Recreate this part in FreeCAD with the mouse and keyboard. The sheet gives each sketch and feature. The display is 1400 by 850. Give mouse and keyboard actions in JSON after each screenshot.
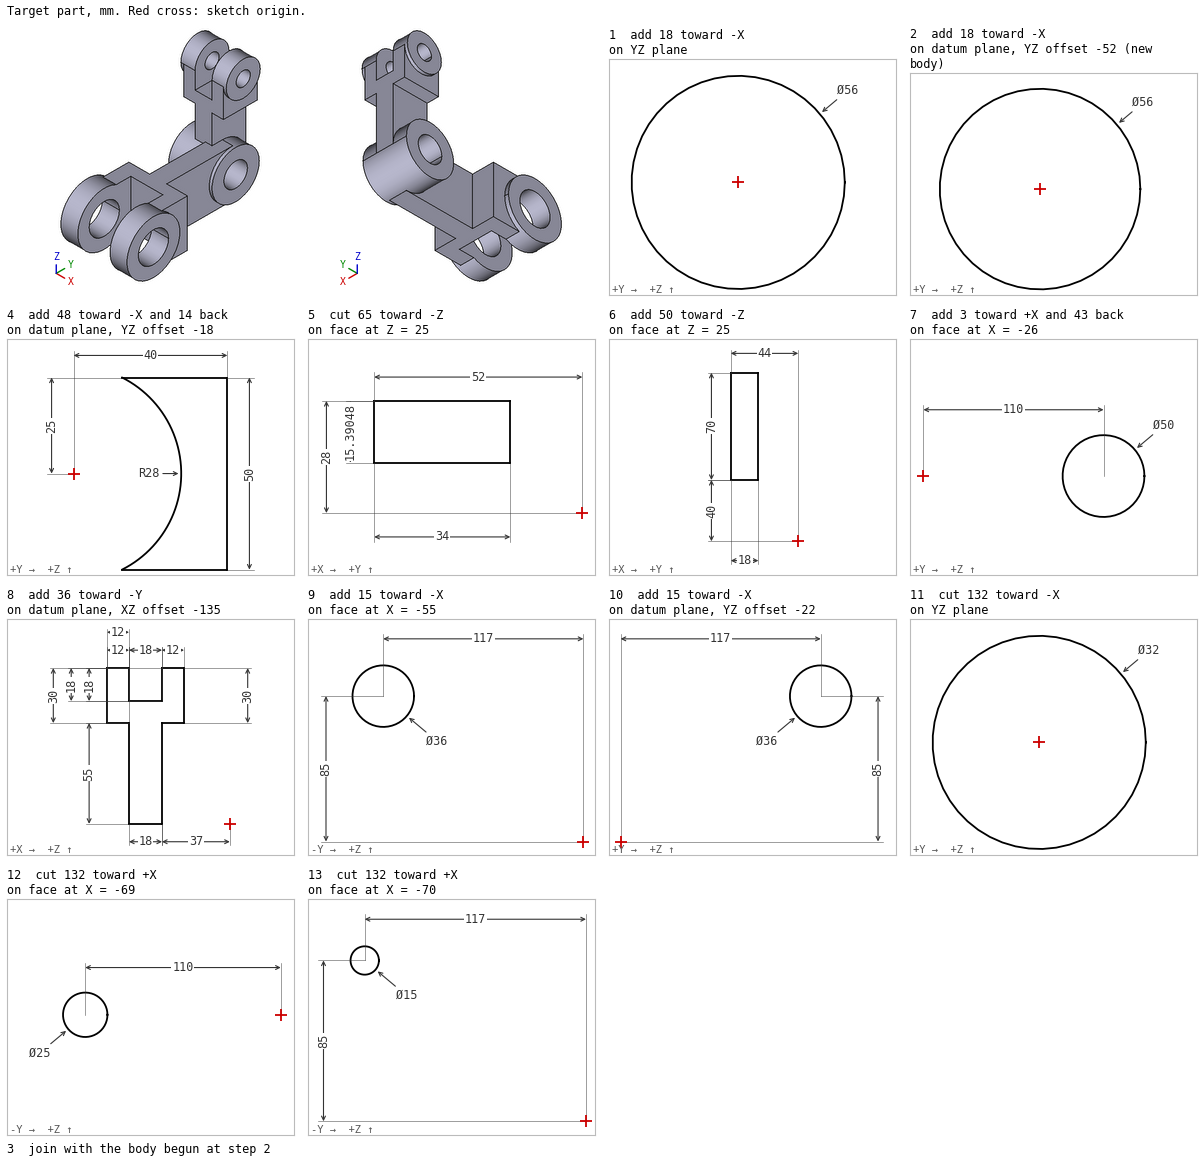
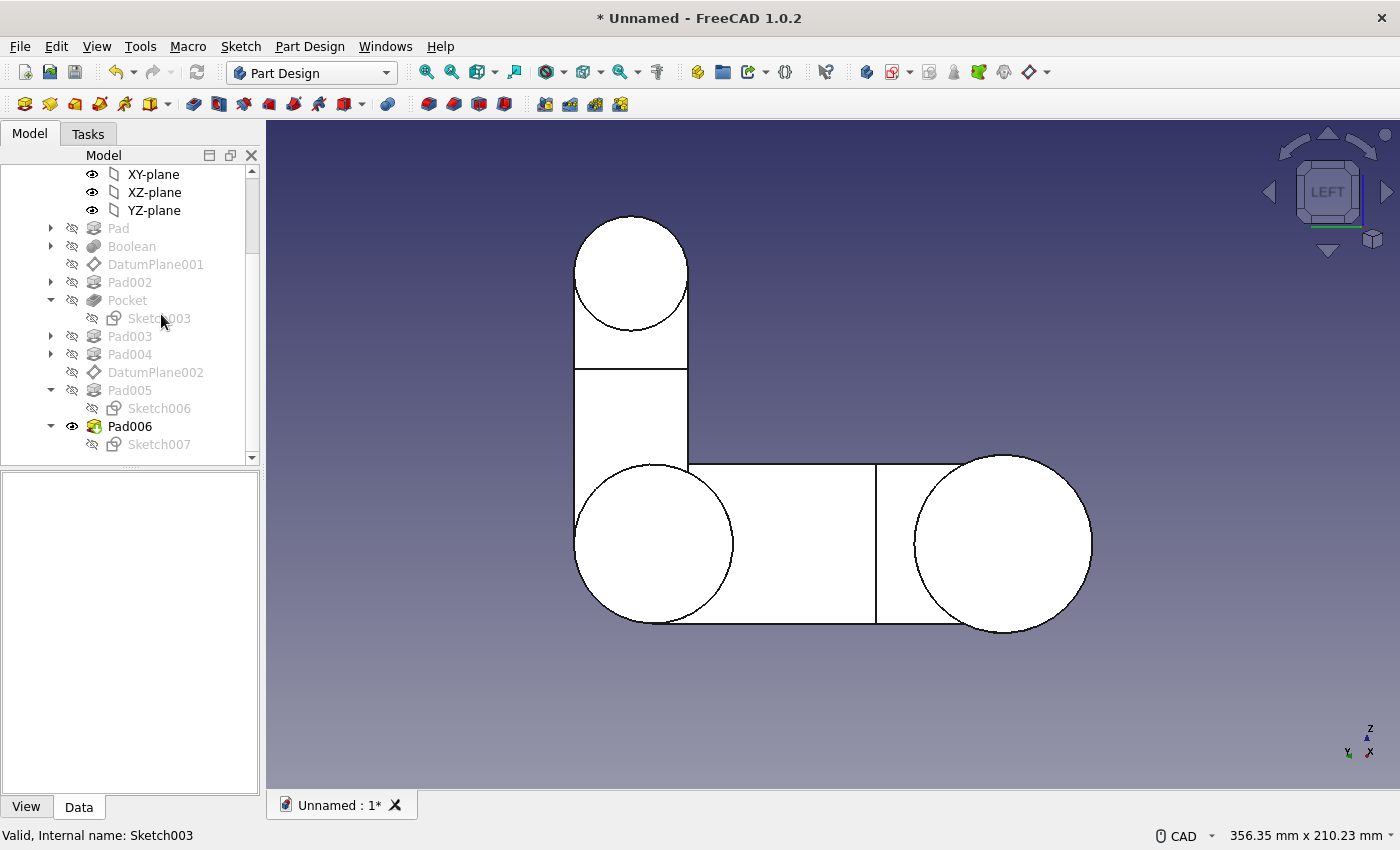
{"action": "scroll", "coordinate": [161, 314], "scroll_direction": "up", "scroll_amount": 15}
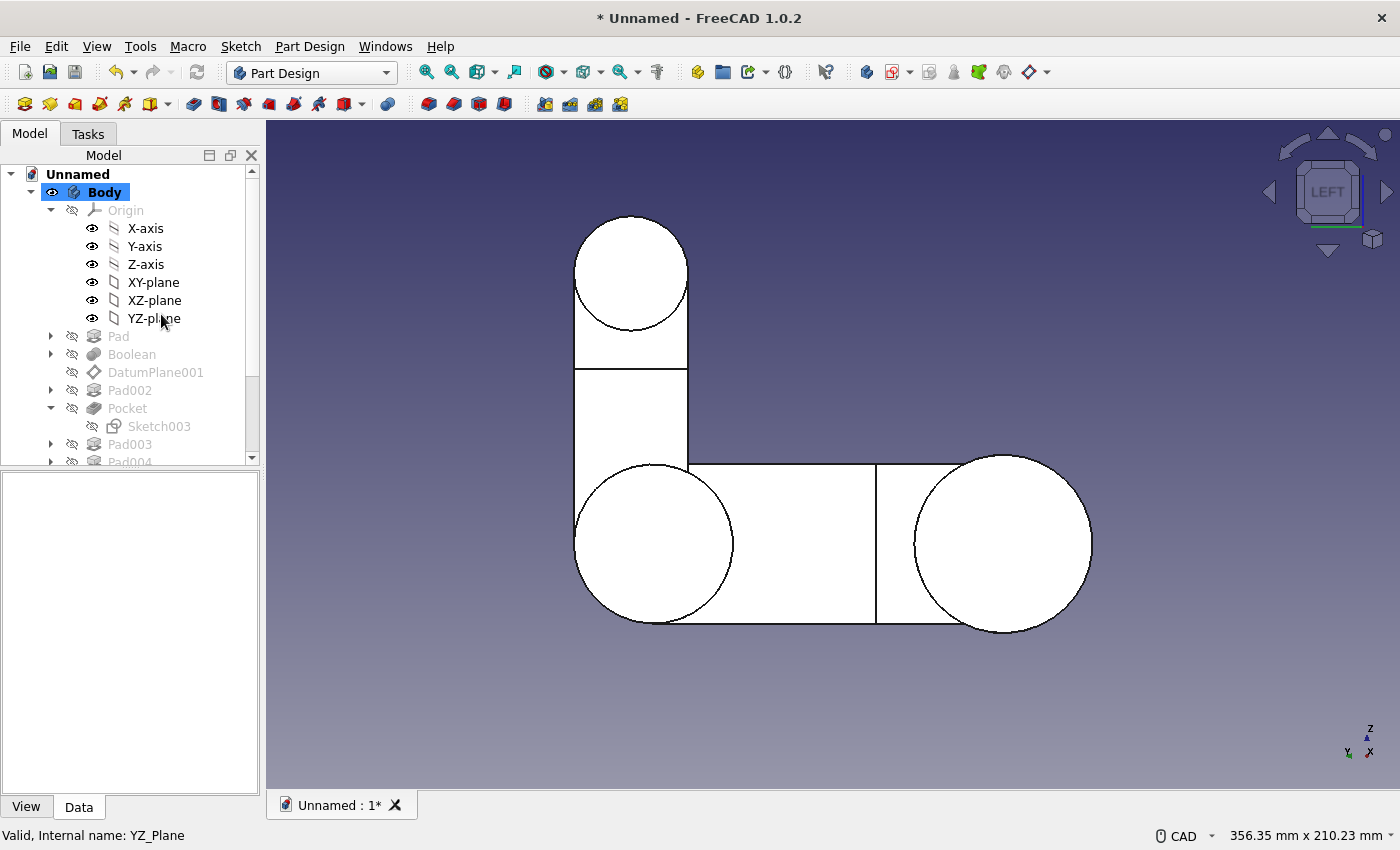
{"action": "left_click", "coordinate": [137, 318]}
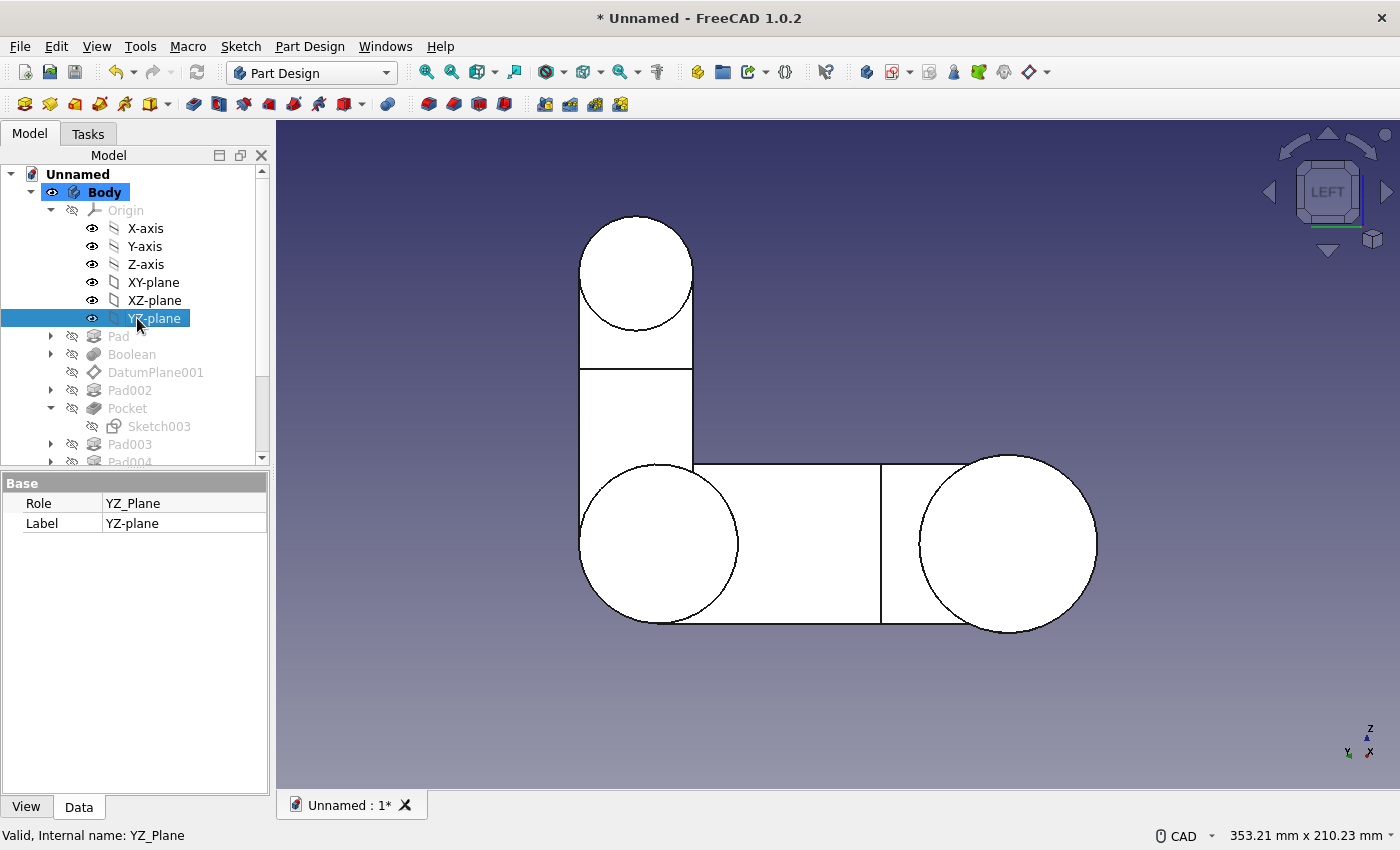
{"action": "left_click", "coordinate": [1028, 72]}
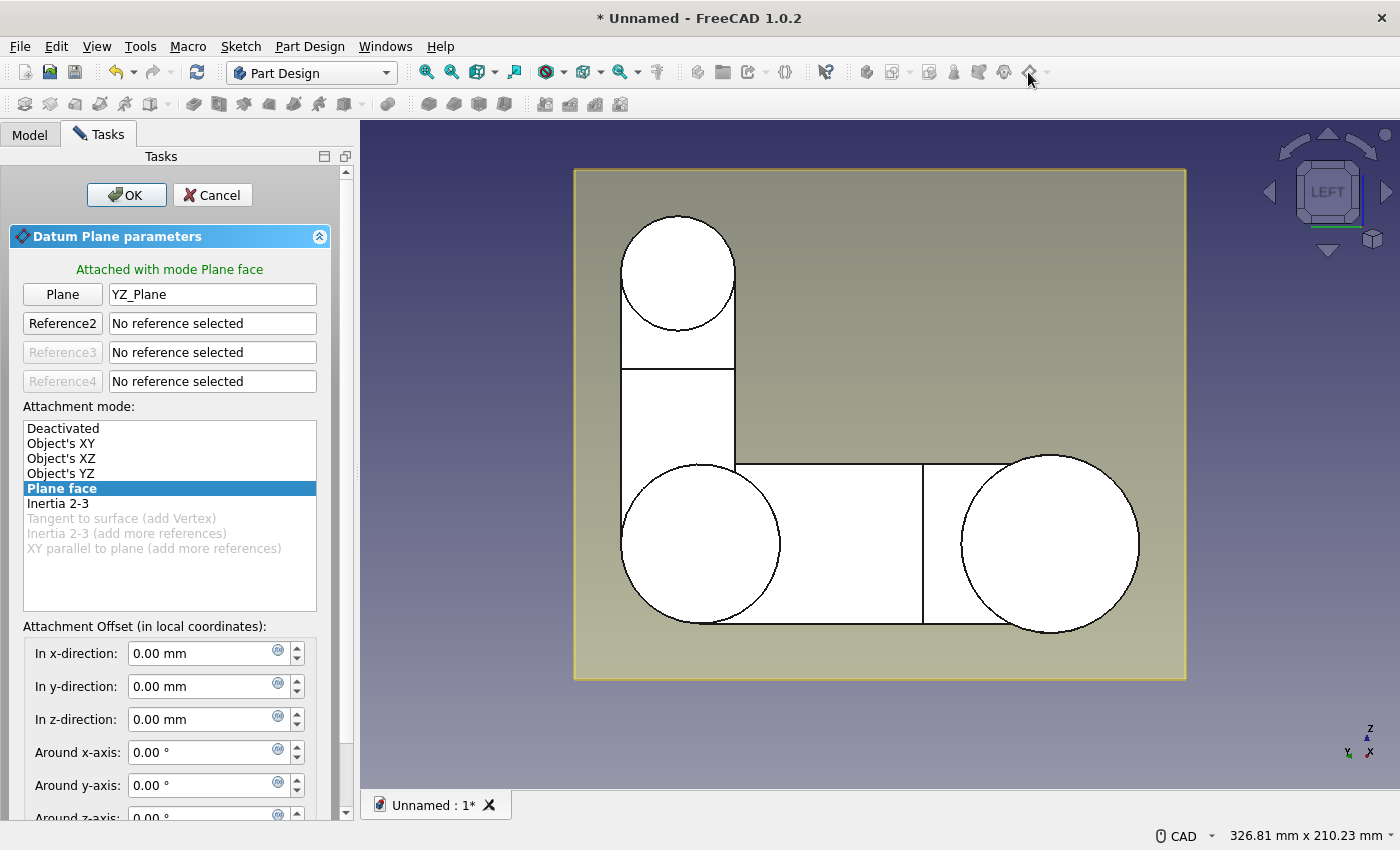
{"action": "triple_click", "coordinate": [210, 720]}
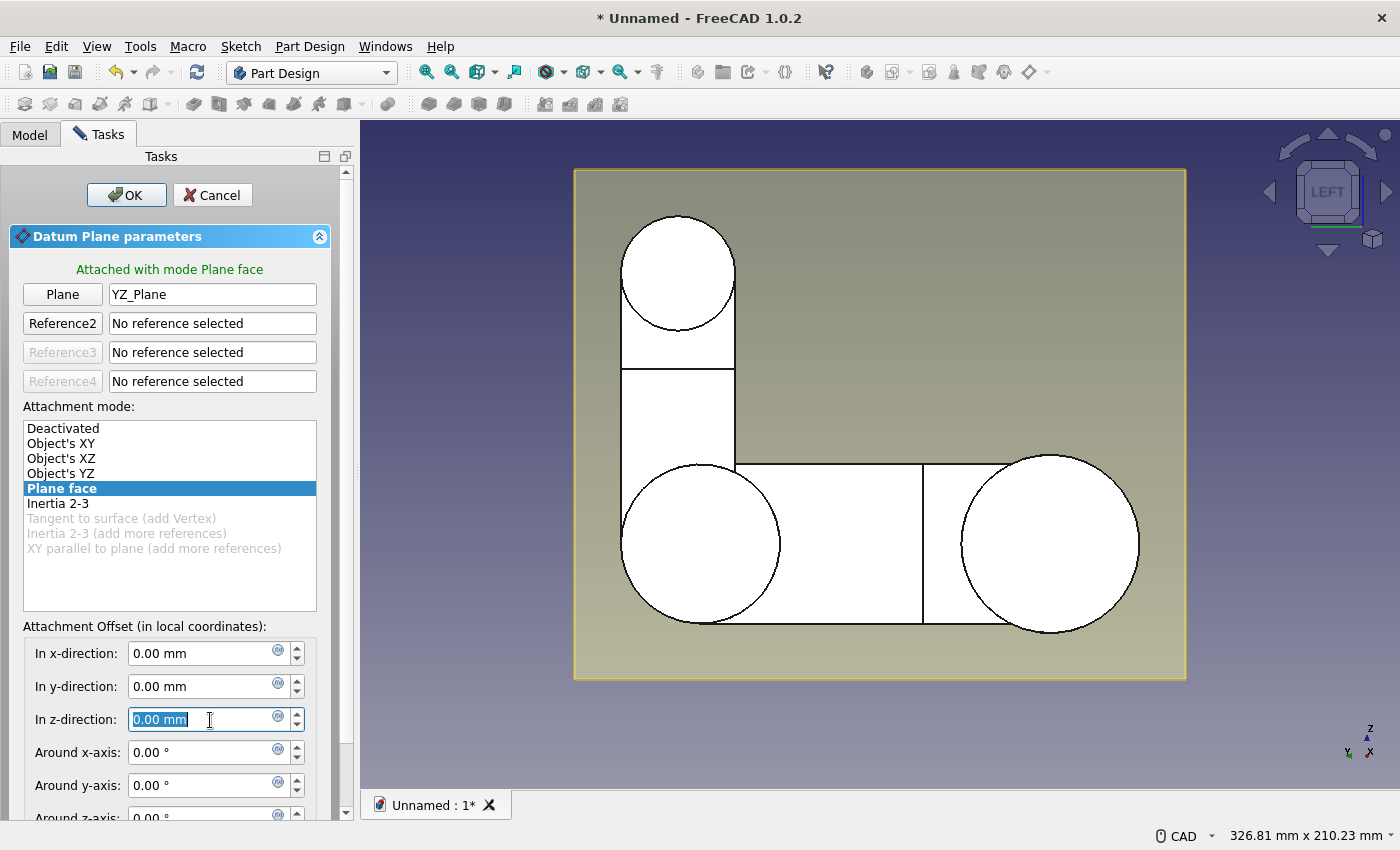
{"action": "type", "text": "-22"}
{"action": "key", "text": "Tab"}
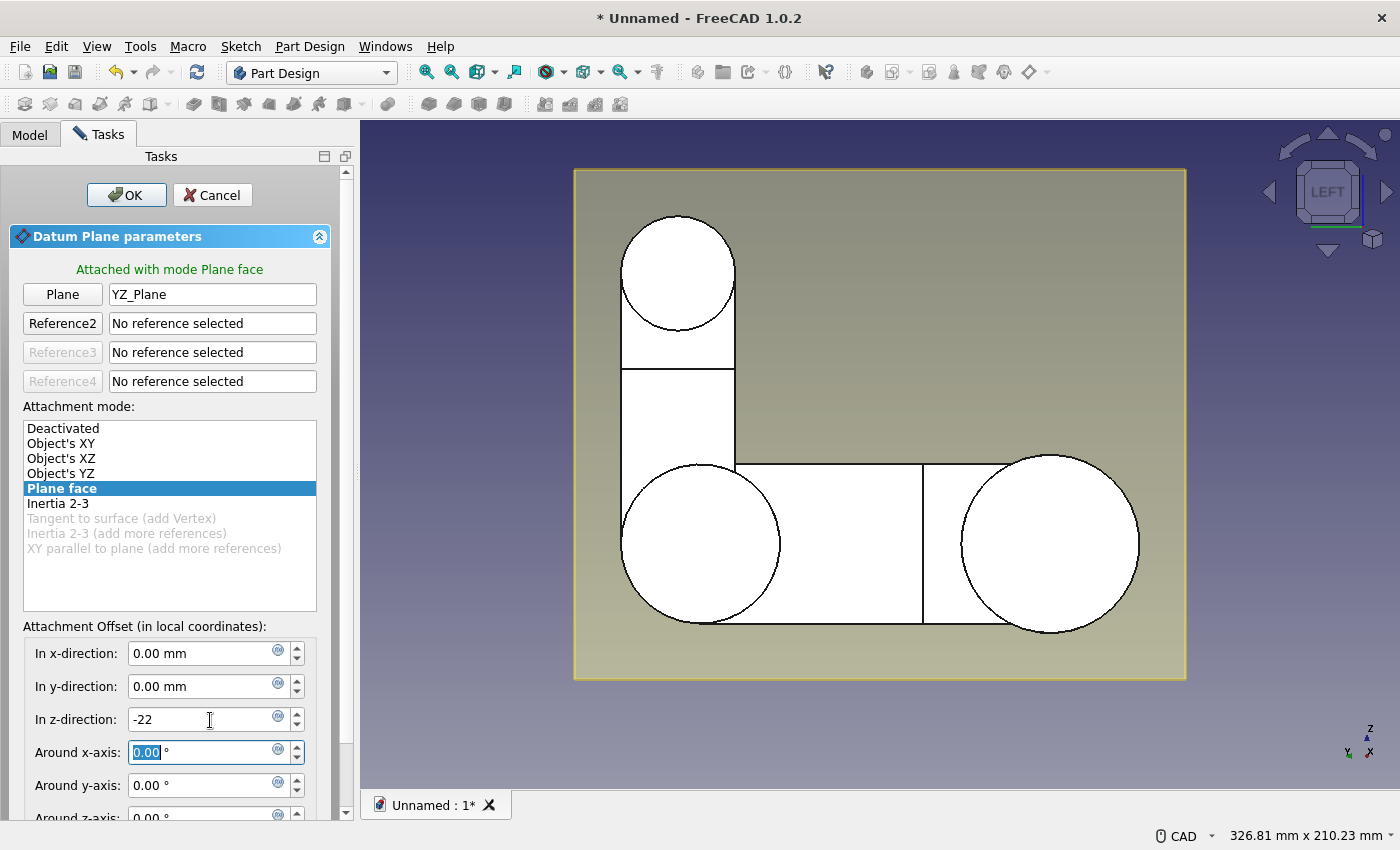
{"action": "left_click", "coordinate": [127, 195]}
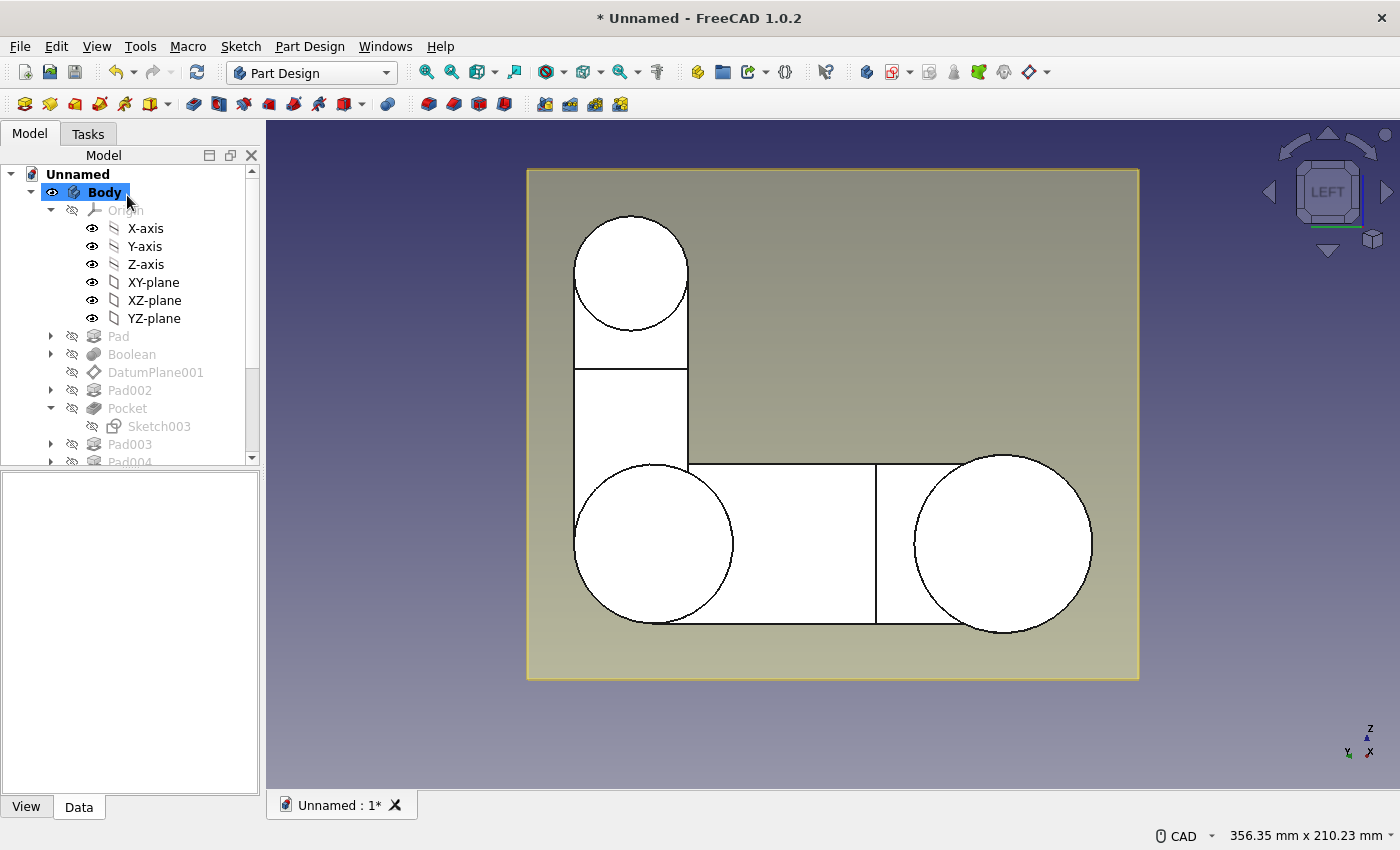
{"action": "scroll", "coordinate": [101, 314], "scroll_direction": "down", "scroll_amount": 3}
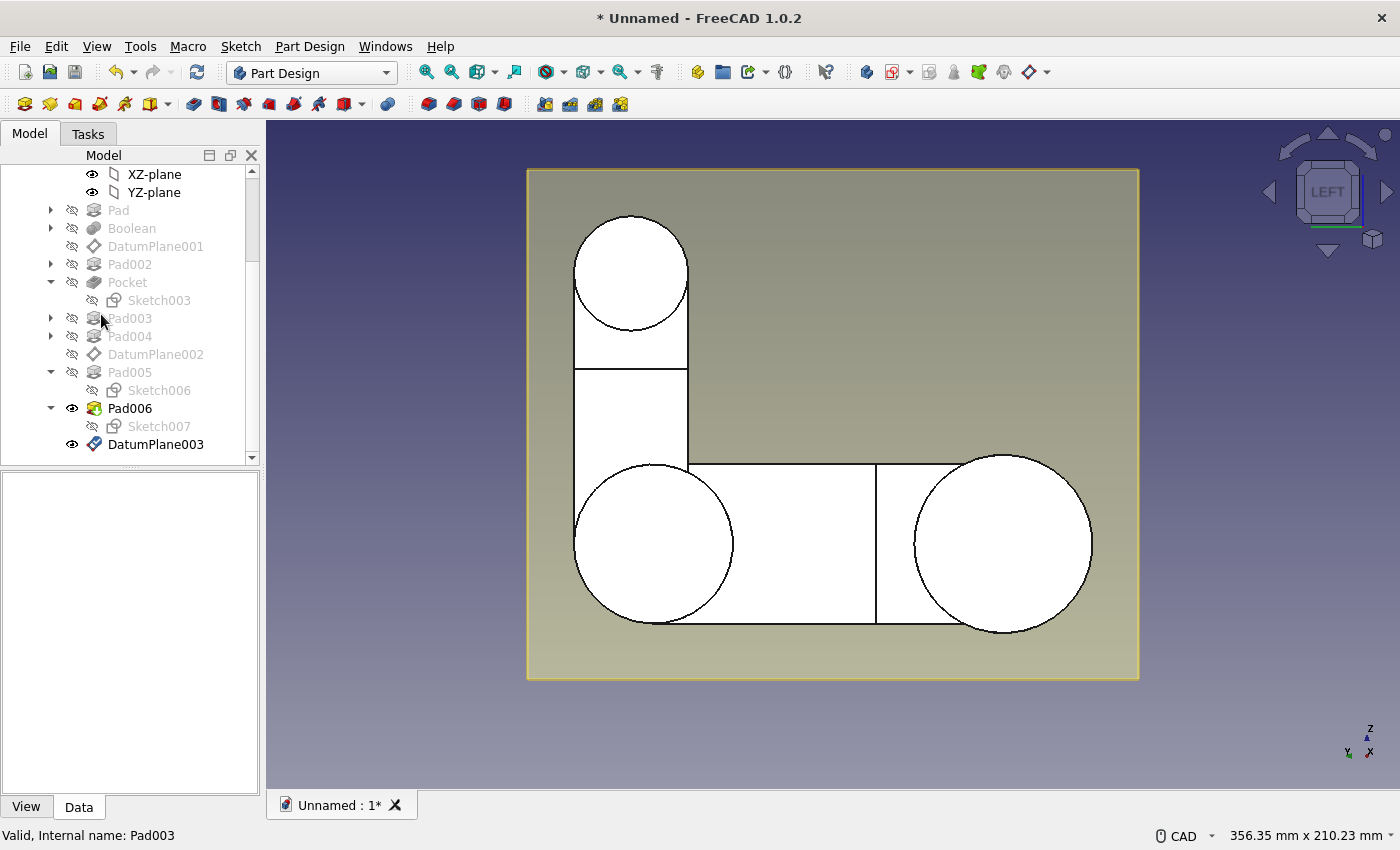
{"action": "left_click", "coordinate": [117, 444]}